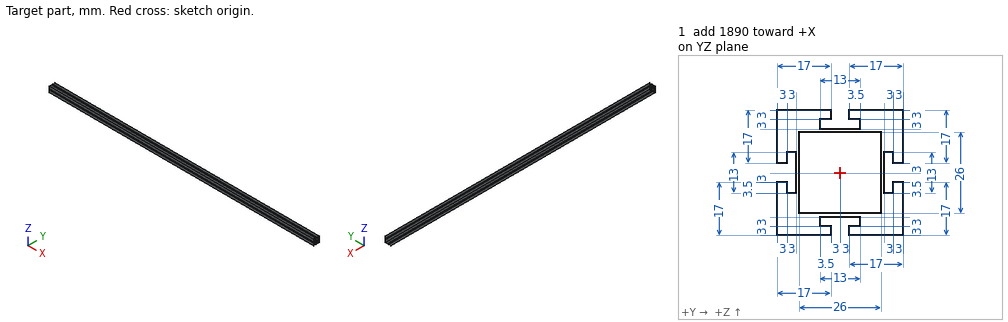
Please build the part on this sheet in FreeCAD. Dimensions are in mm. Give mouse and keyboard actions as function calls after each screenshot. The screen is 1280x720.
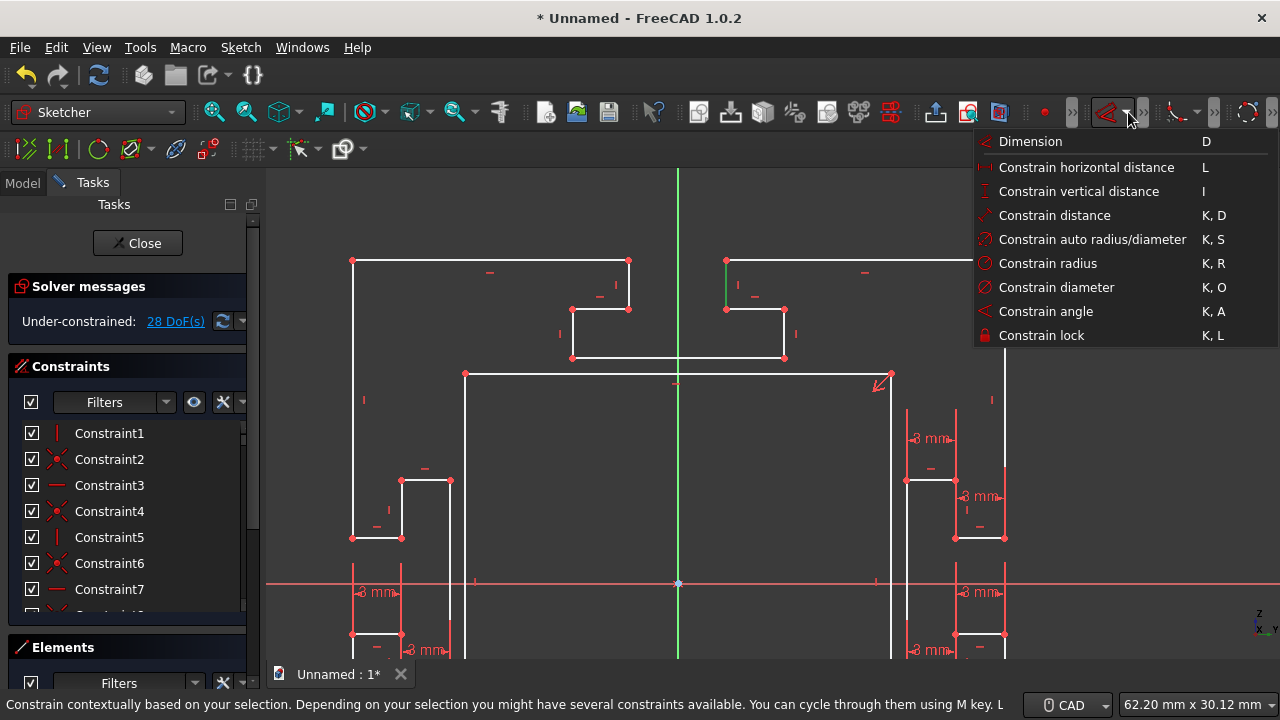
click(1126, 191)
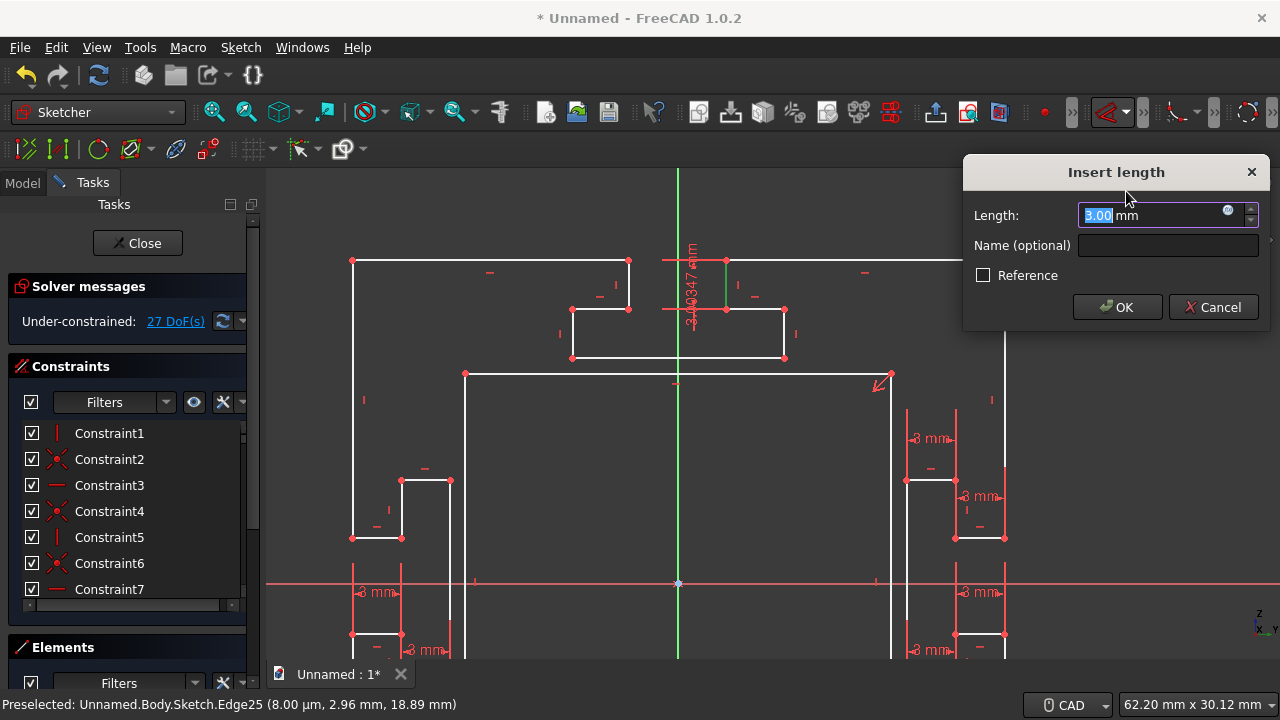
text(3)
key(Return)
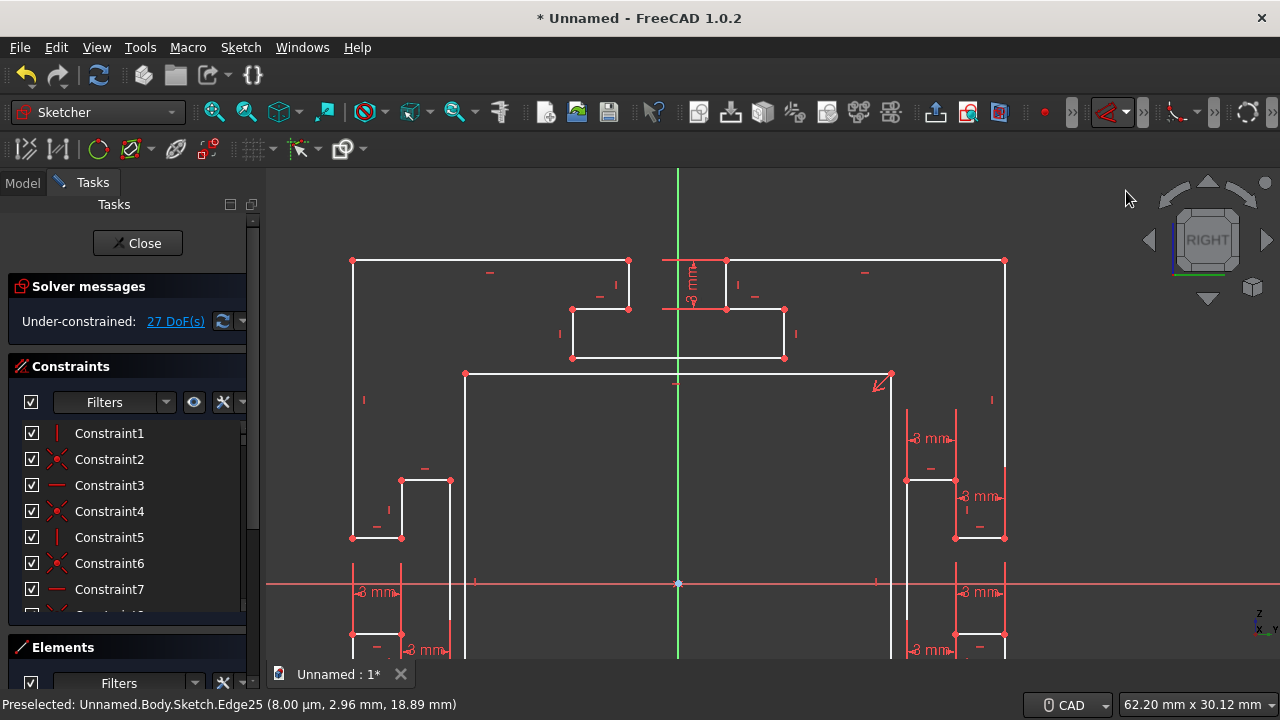
click(784, 324)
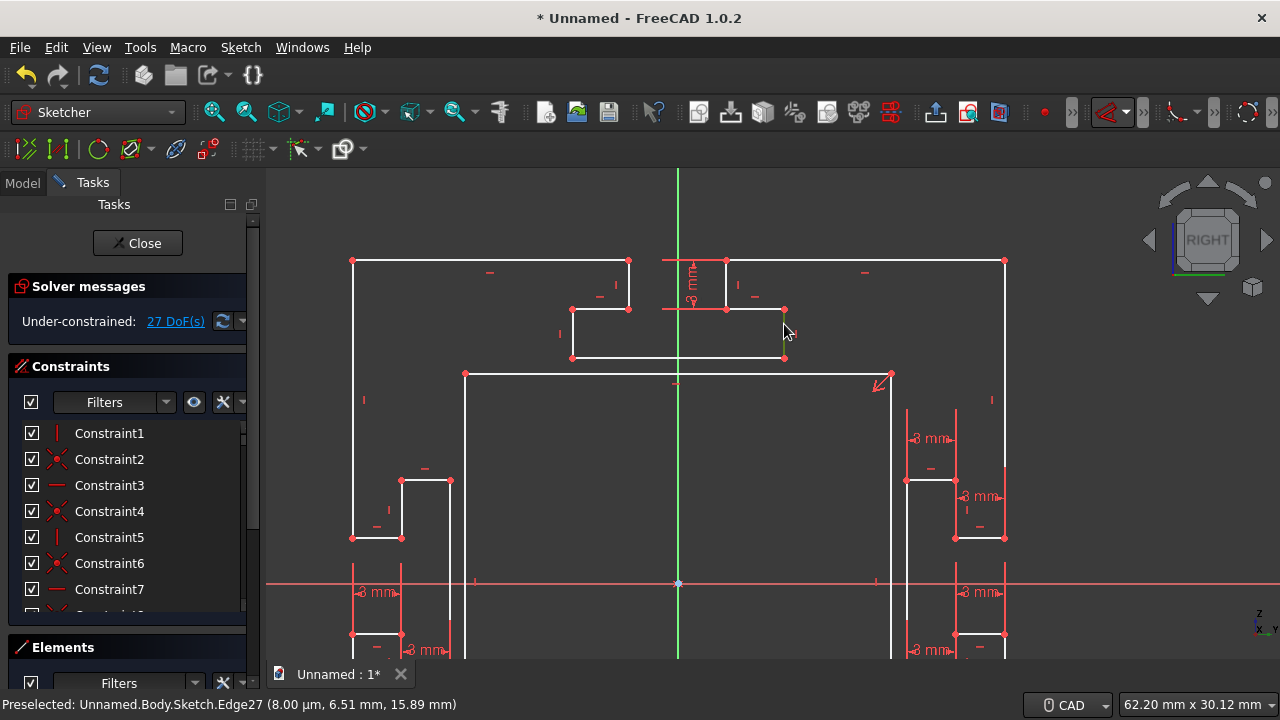
key(i)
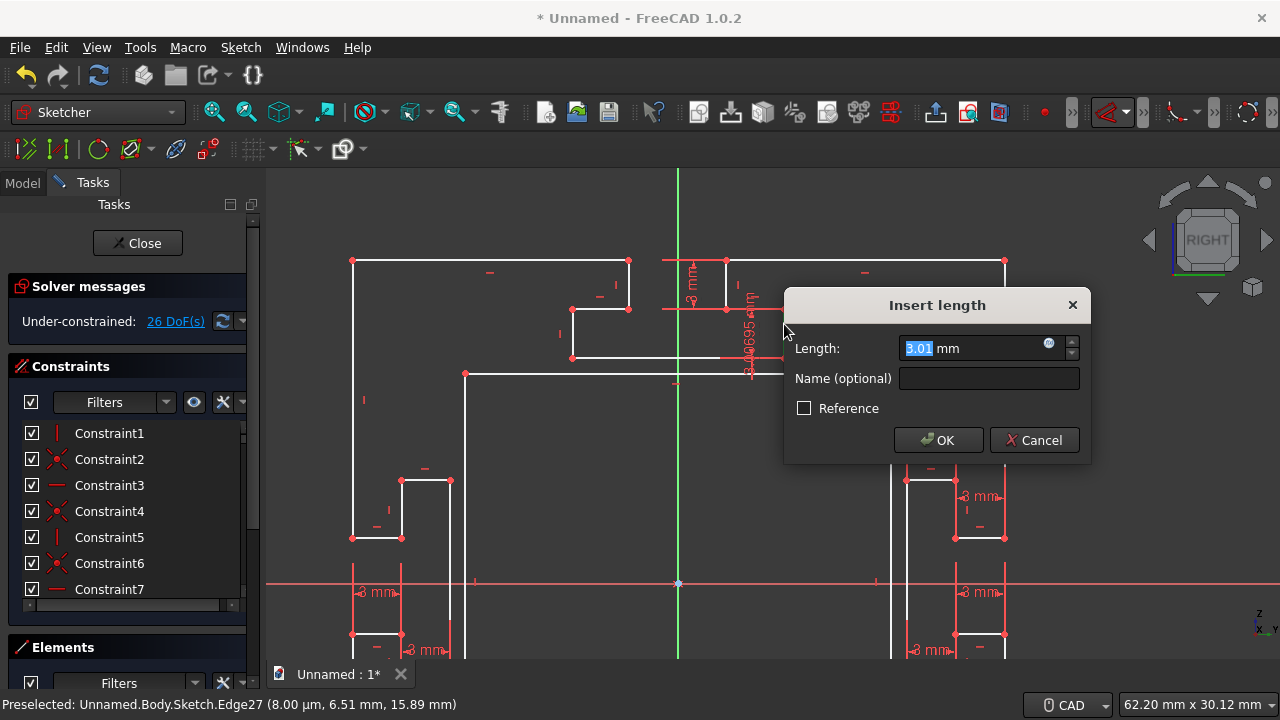
text(3)
key(Return)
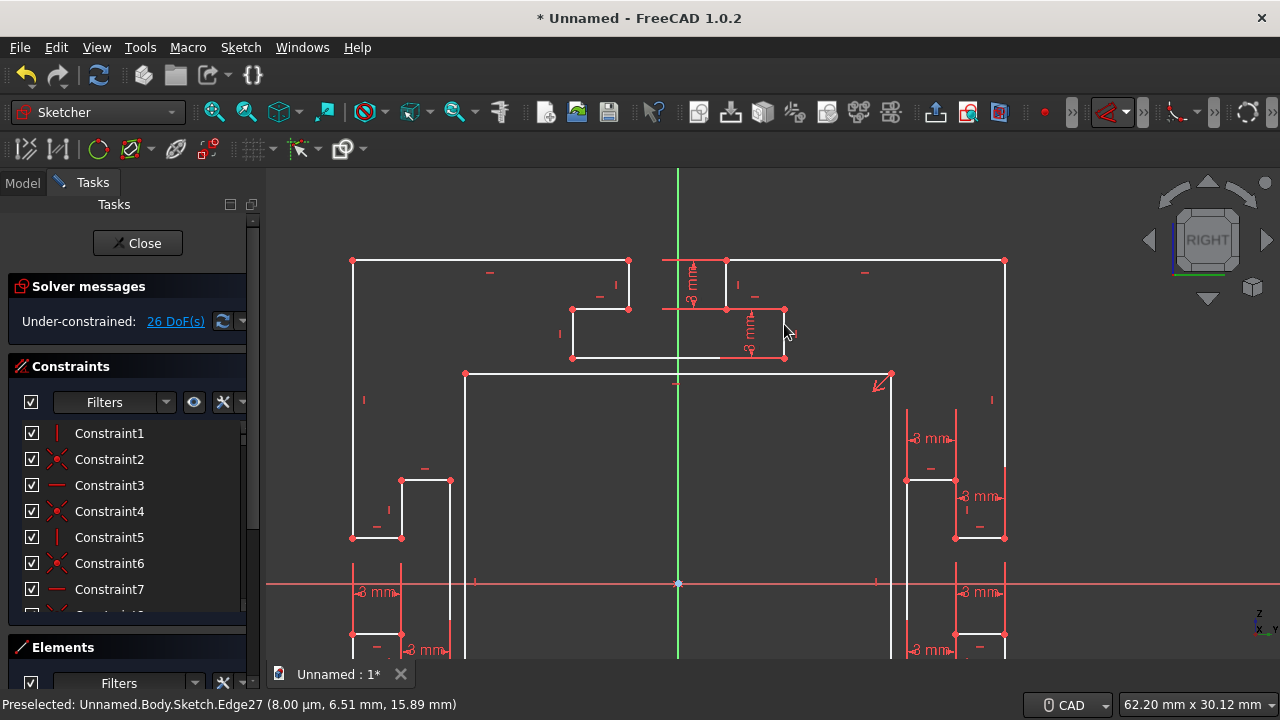
click(573, 343)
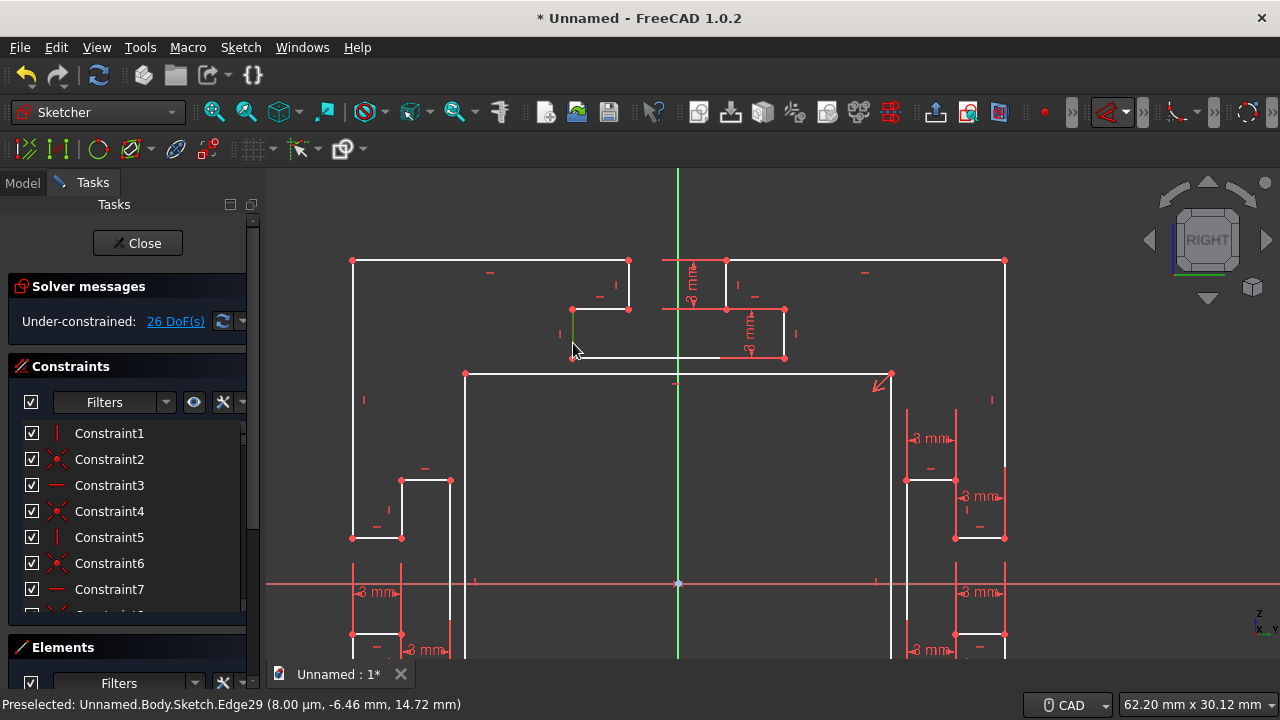
key(i)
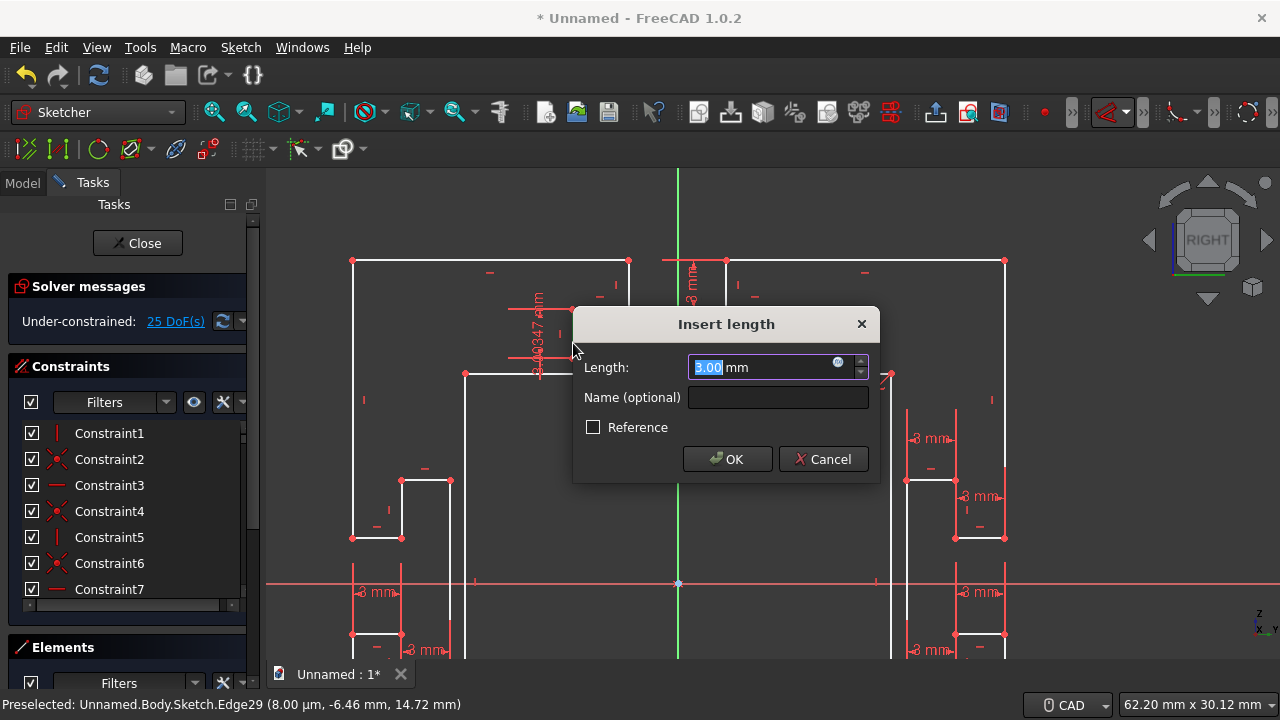
text(3)
key(Return)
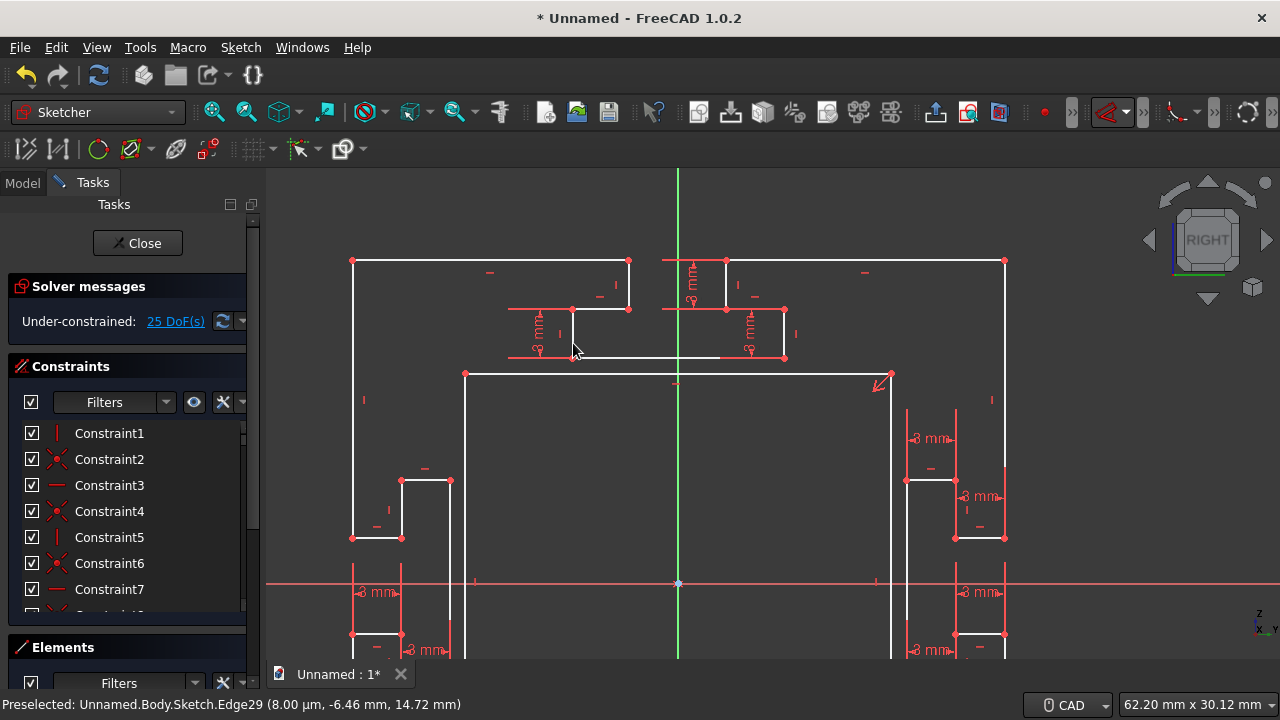
click(629, 294)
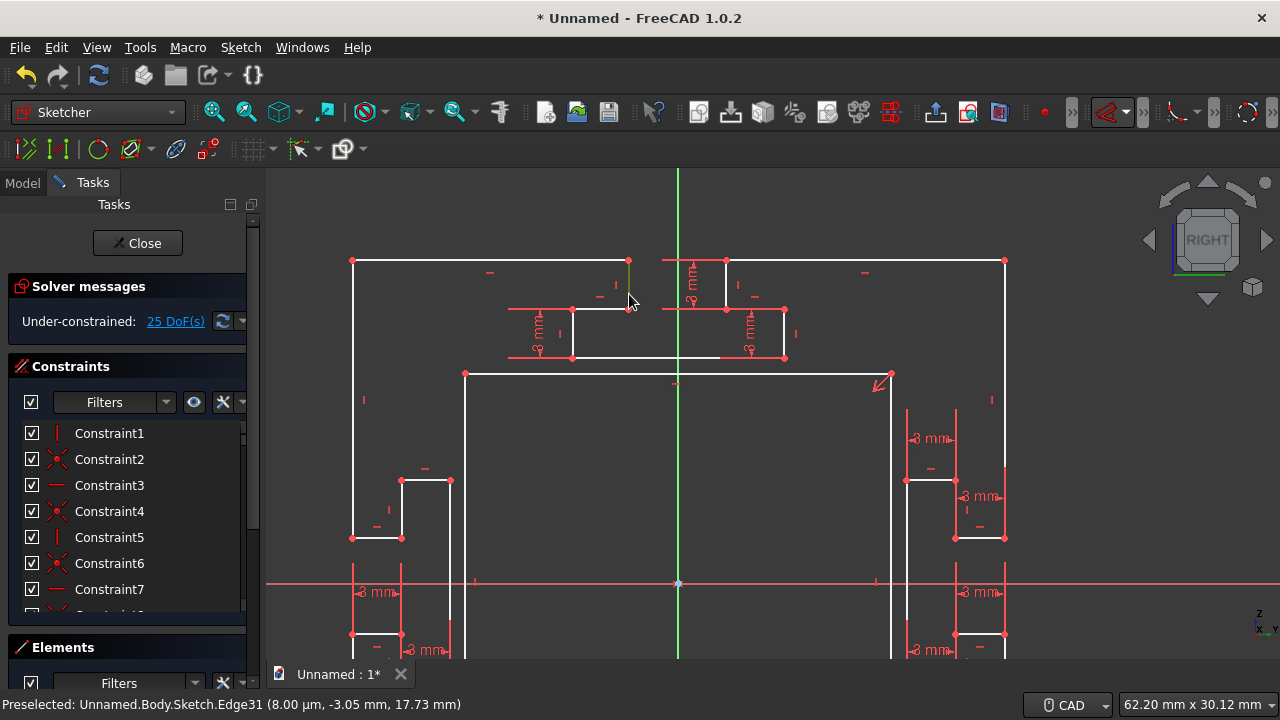
key(i)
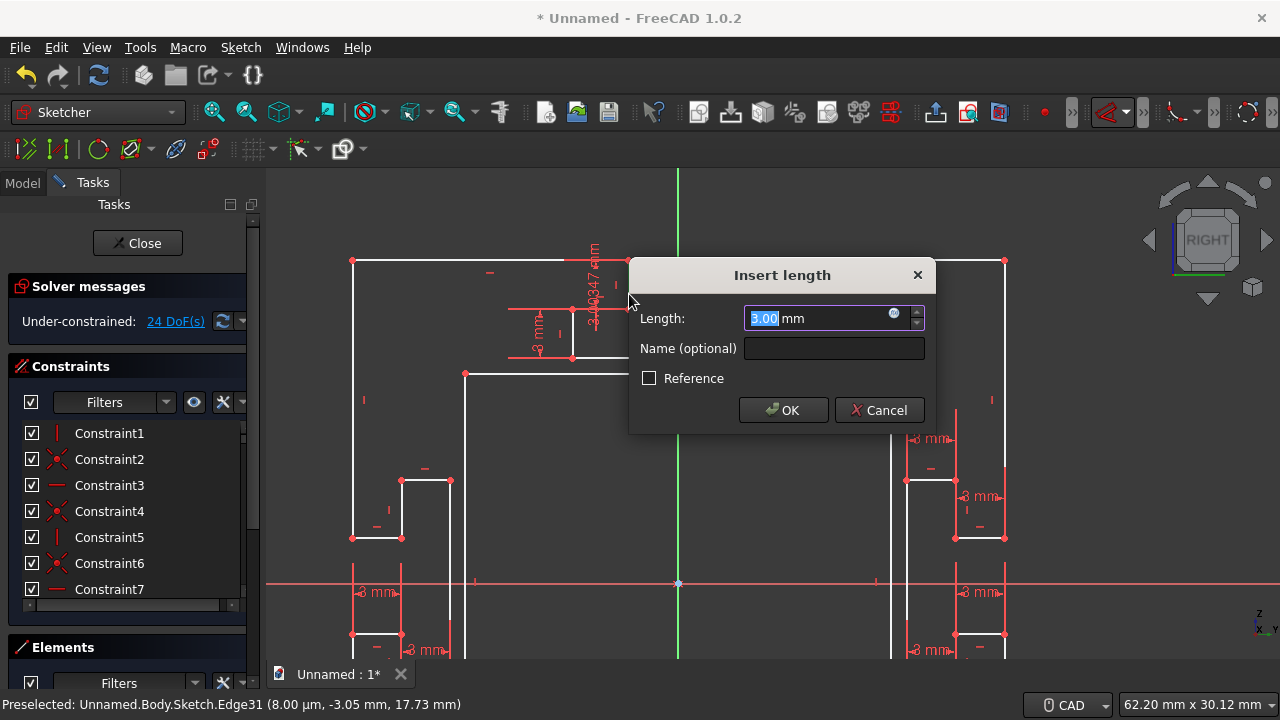
text(3)
key(Return)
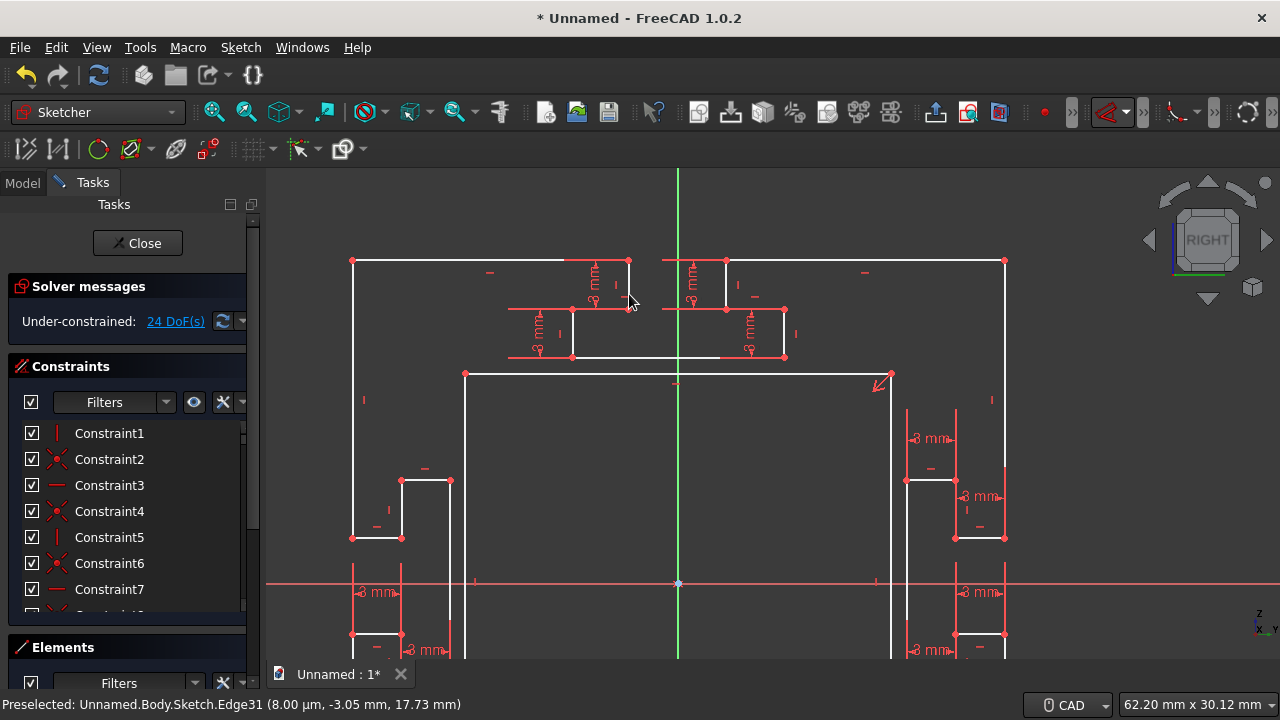
click(367, 538)